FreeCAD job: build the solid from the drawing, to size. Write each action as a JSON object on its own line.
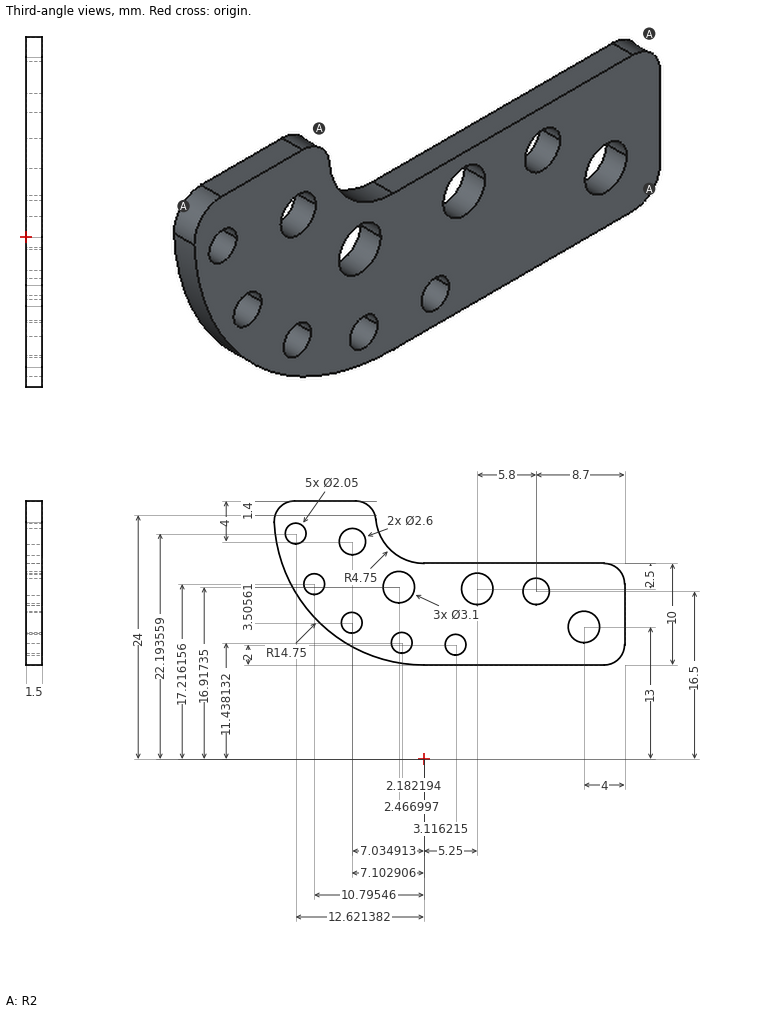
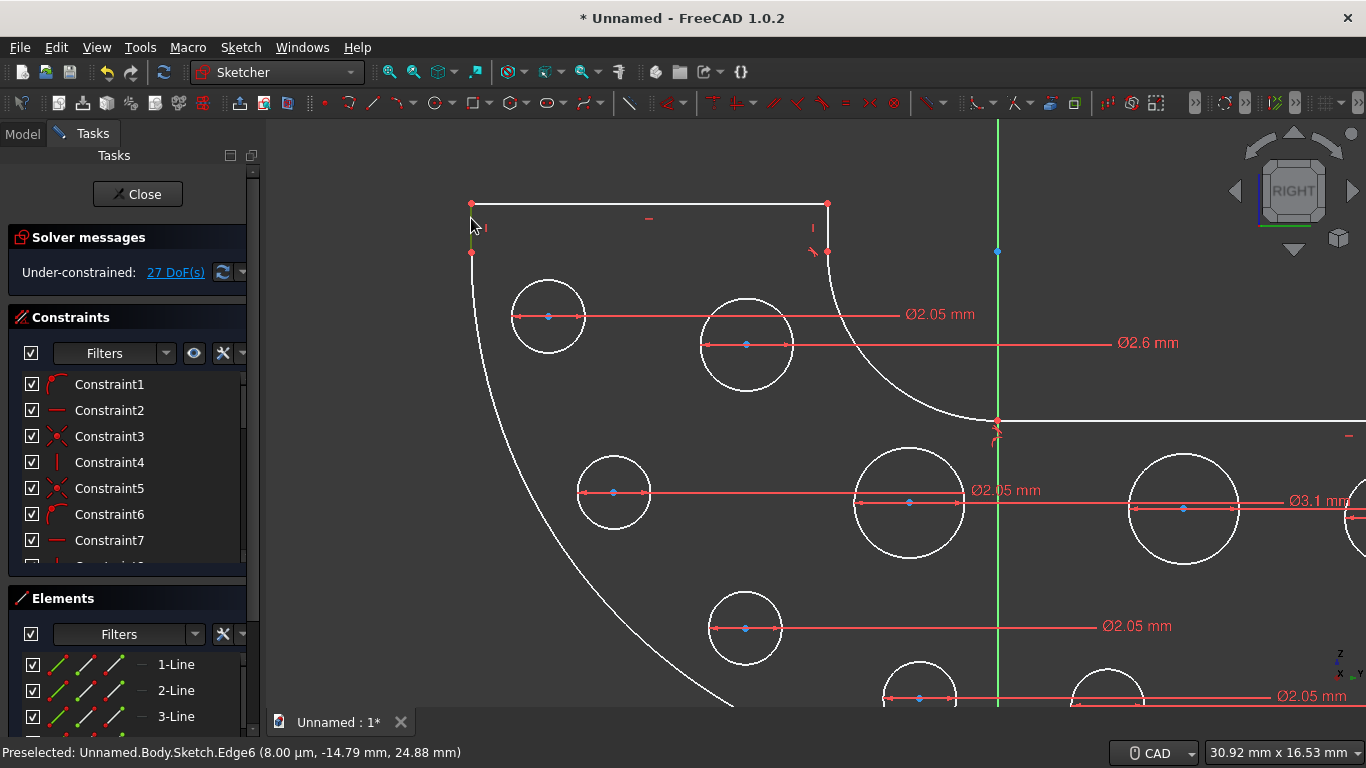
{"action": "left_click", "coordinate": [529, 491]}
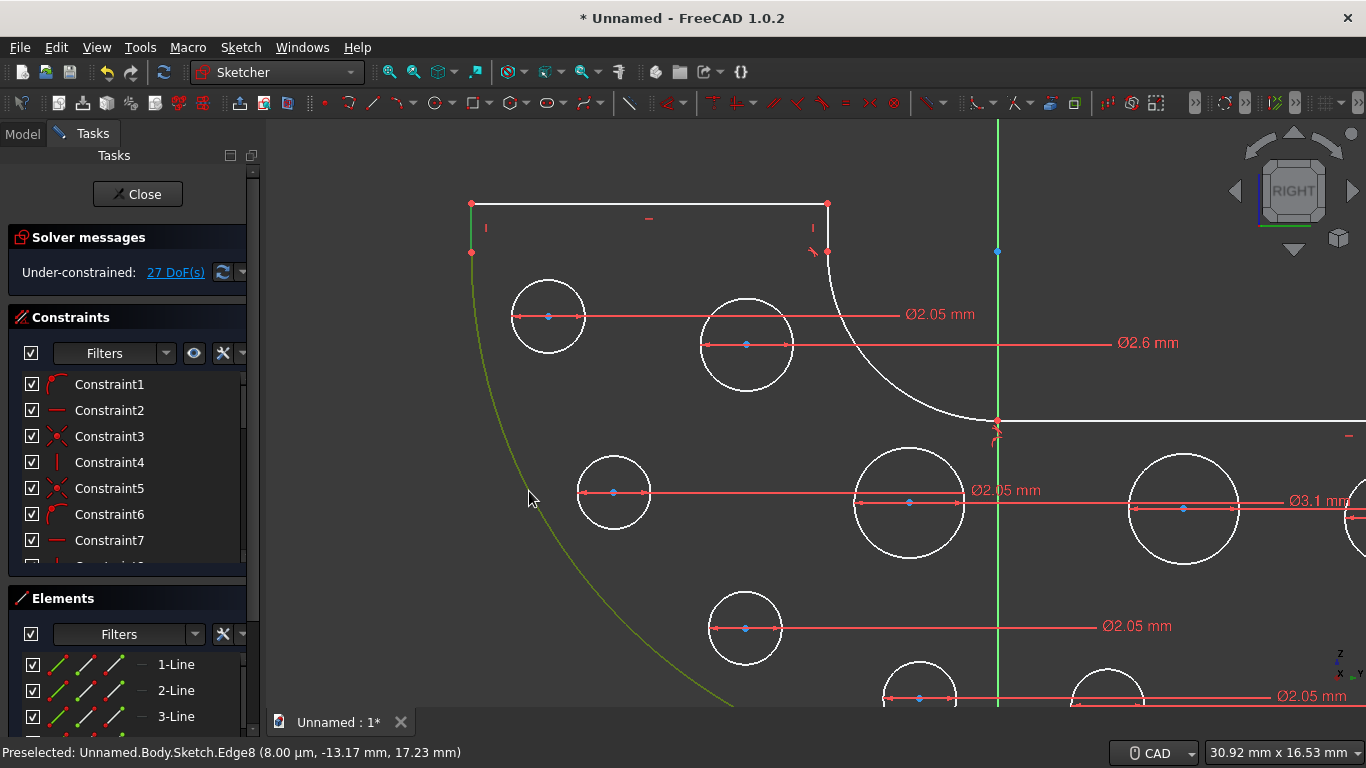
{"action": "left_click", "coordinate": [822, 104]}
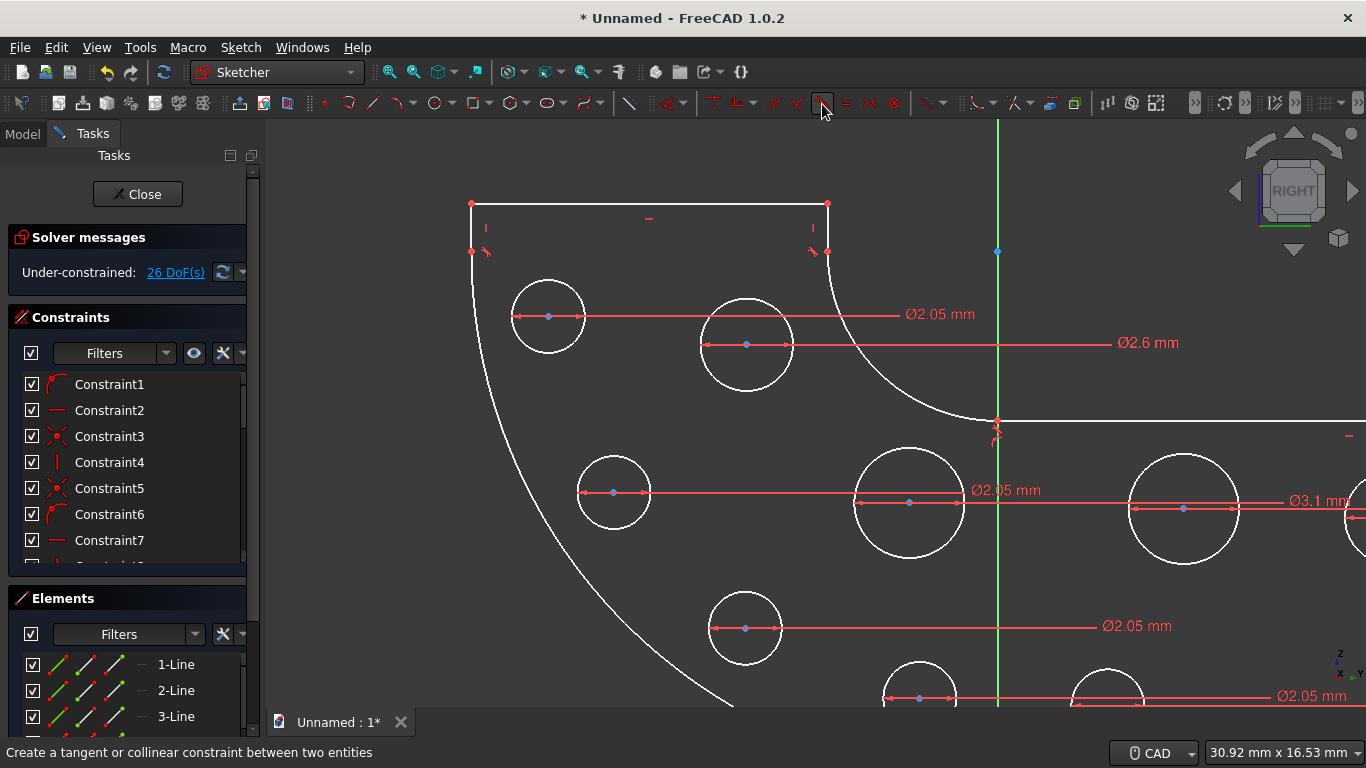
{"action": "left_click", "coordinate": [668, 104]}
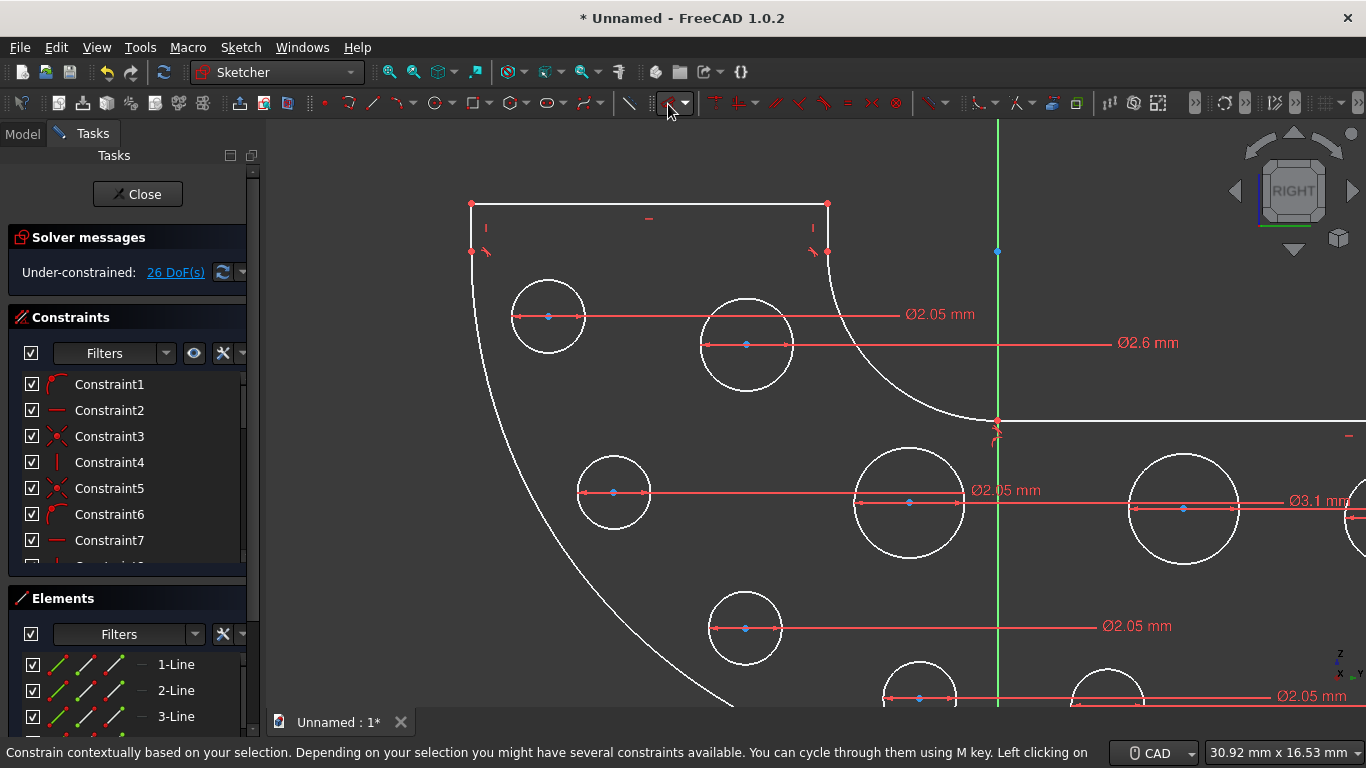
{"action": "left_click", "coordinate": [846, 328]}
{"action": "left_click", "coordinate": [817, 342]}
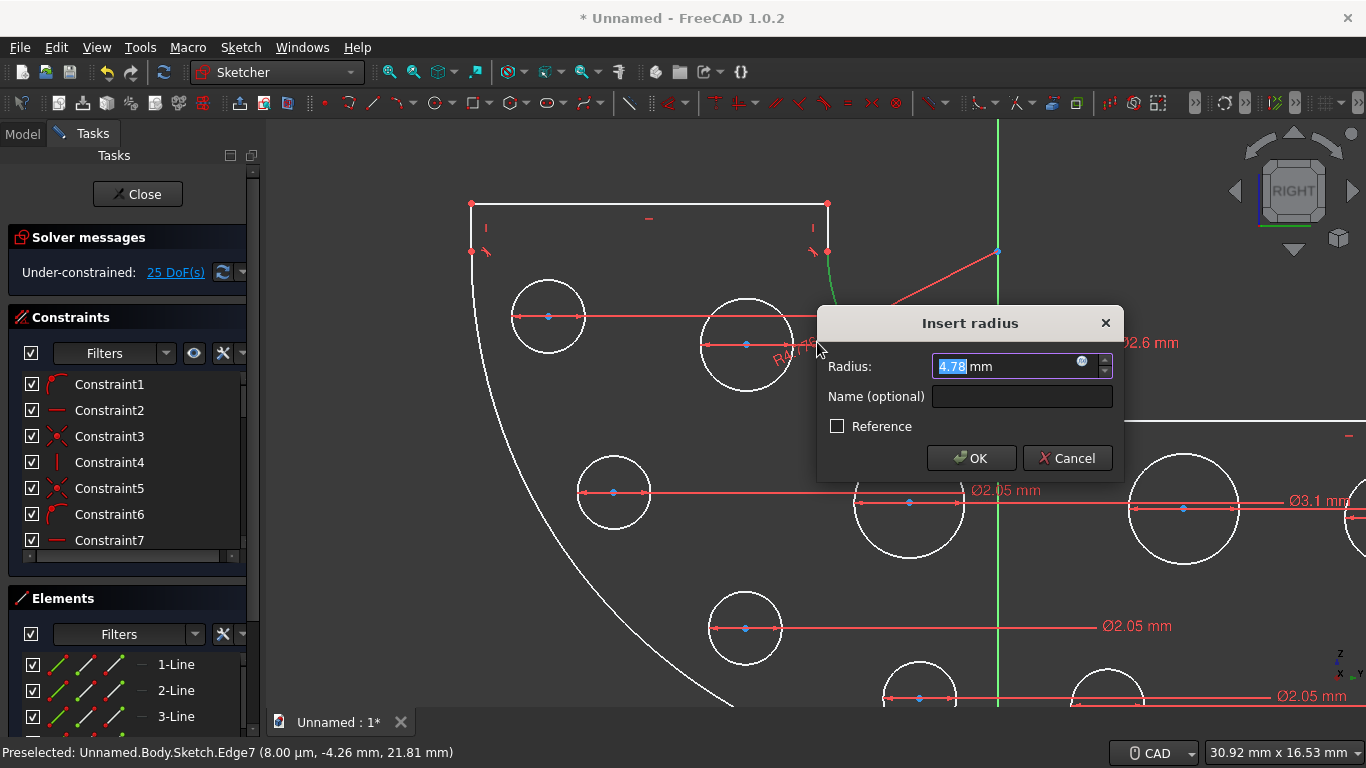
{"action": "type", "text": "4.75"}
{"action": "key", "text": "Return"}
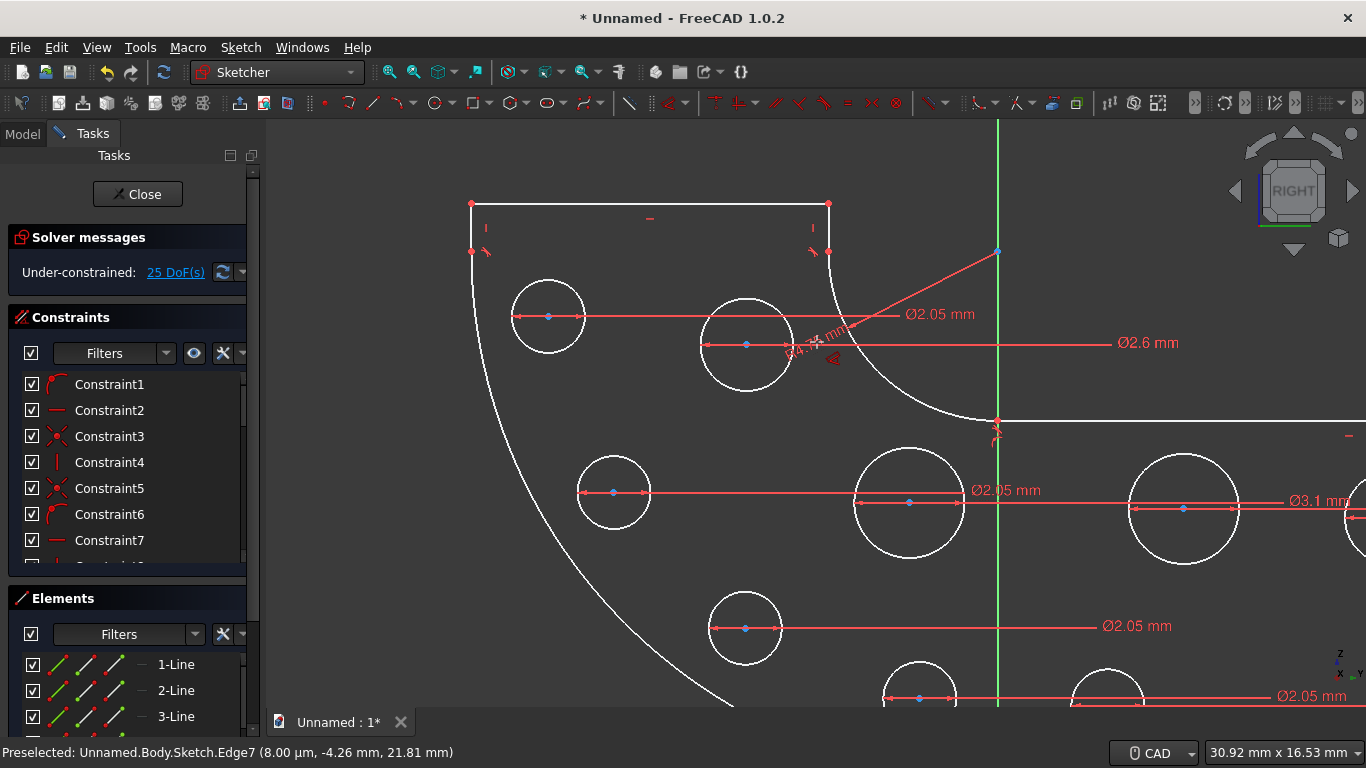
{"action": "left_click", "coordinate": [529, 491]}
{"action": "left_click", "coordinate": [500, 506]}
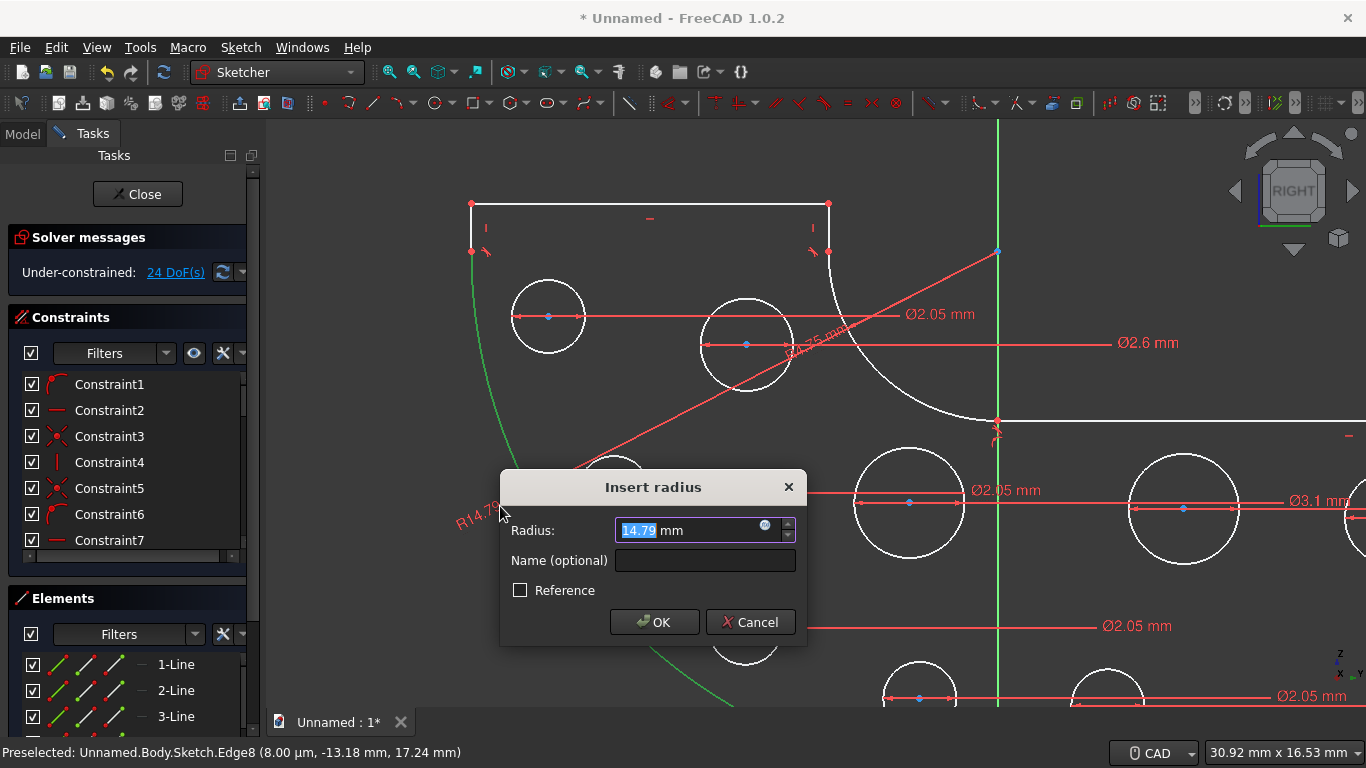
{"action": "type", "text": "14.75"}
{"action": "key", "text": "Return"}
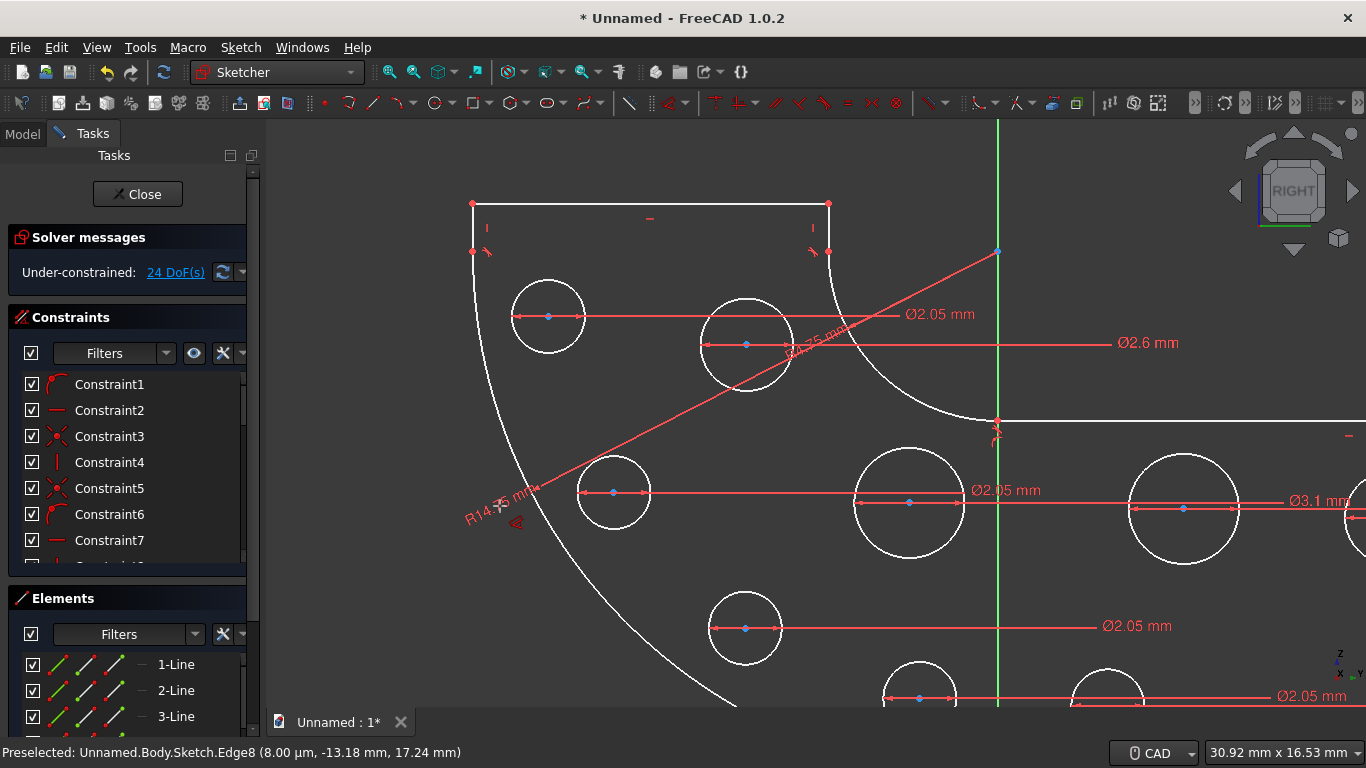
{"action": "scroll", "coordinate": [471, 218], "scroll_direction": "down", "scroll_amount": 4}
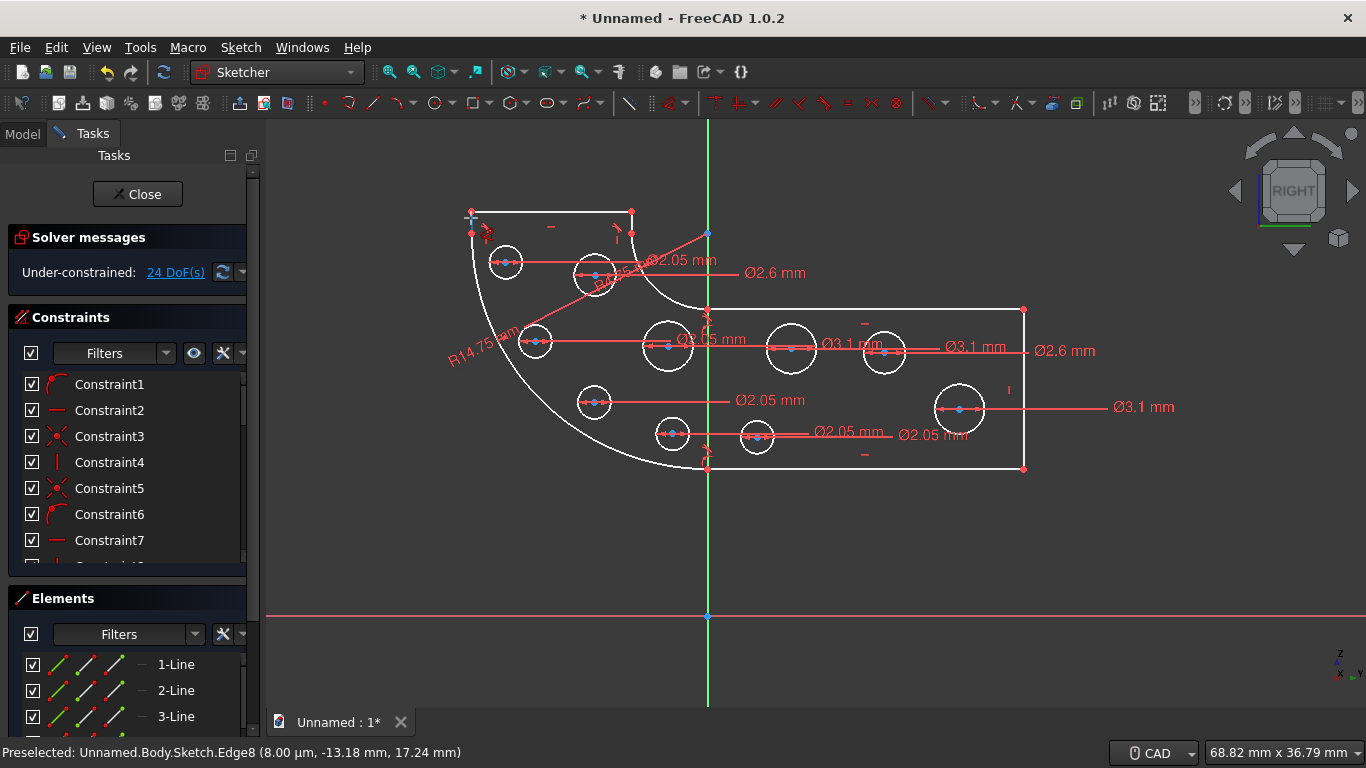
{"action": "left_click", "coordinate": [1024, 421]}
{"action": "left_click", "coordinate": [1058, 389]}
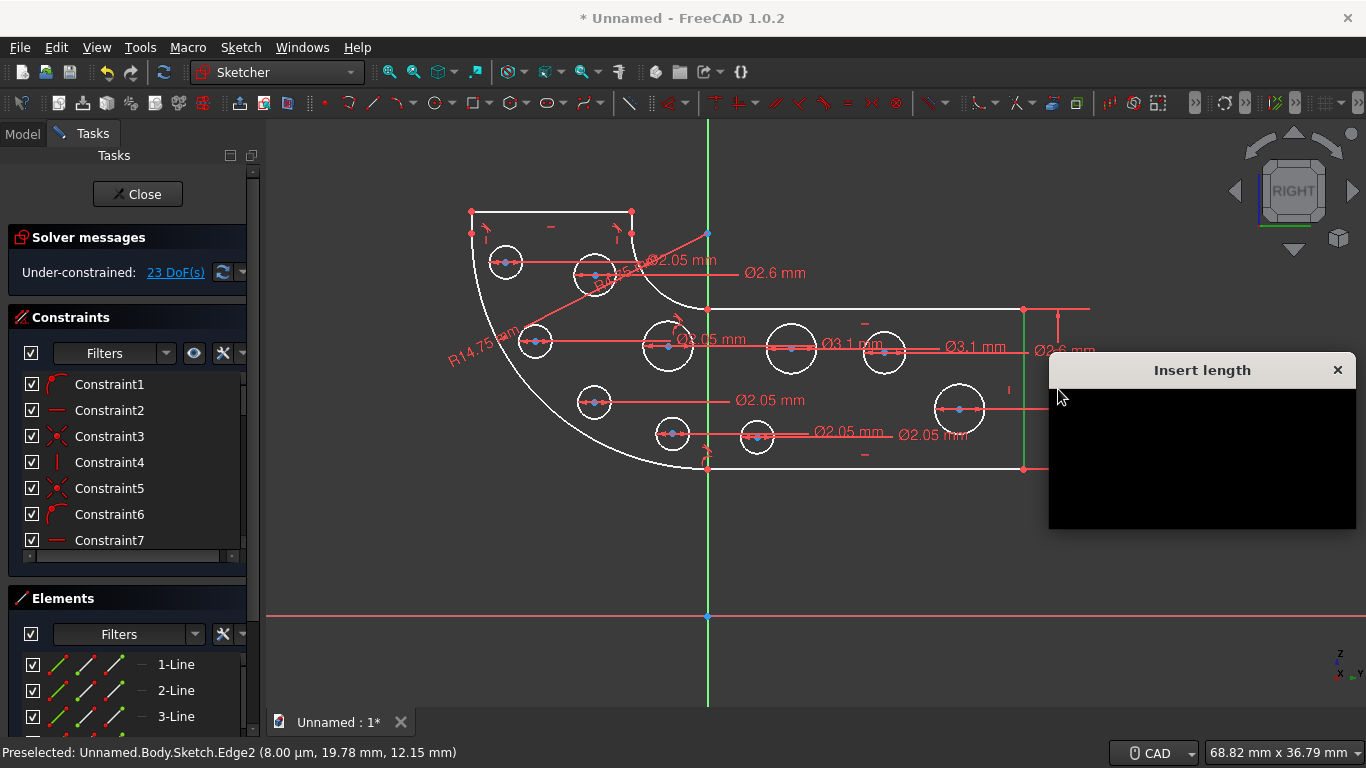
{"action": "type", "text": "10"}
{"action": "key", "text": "Return"}